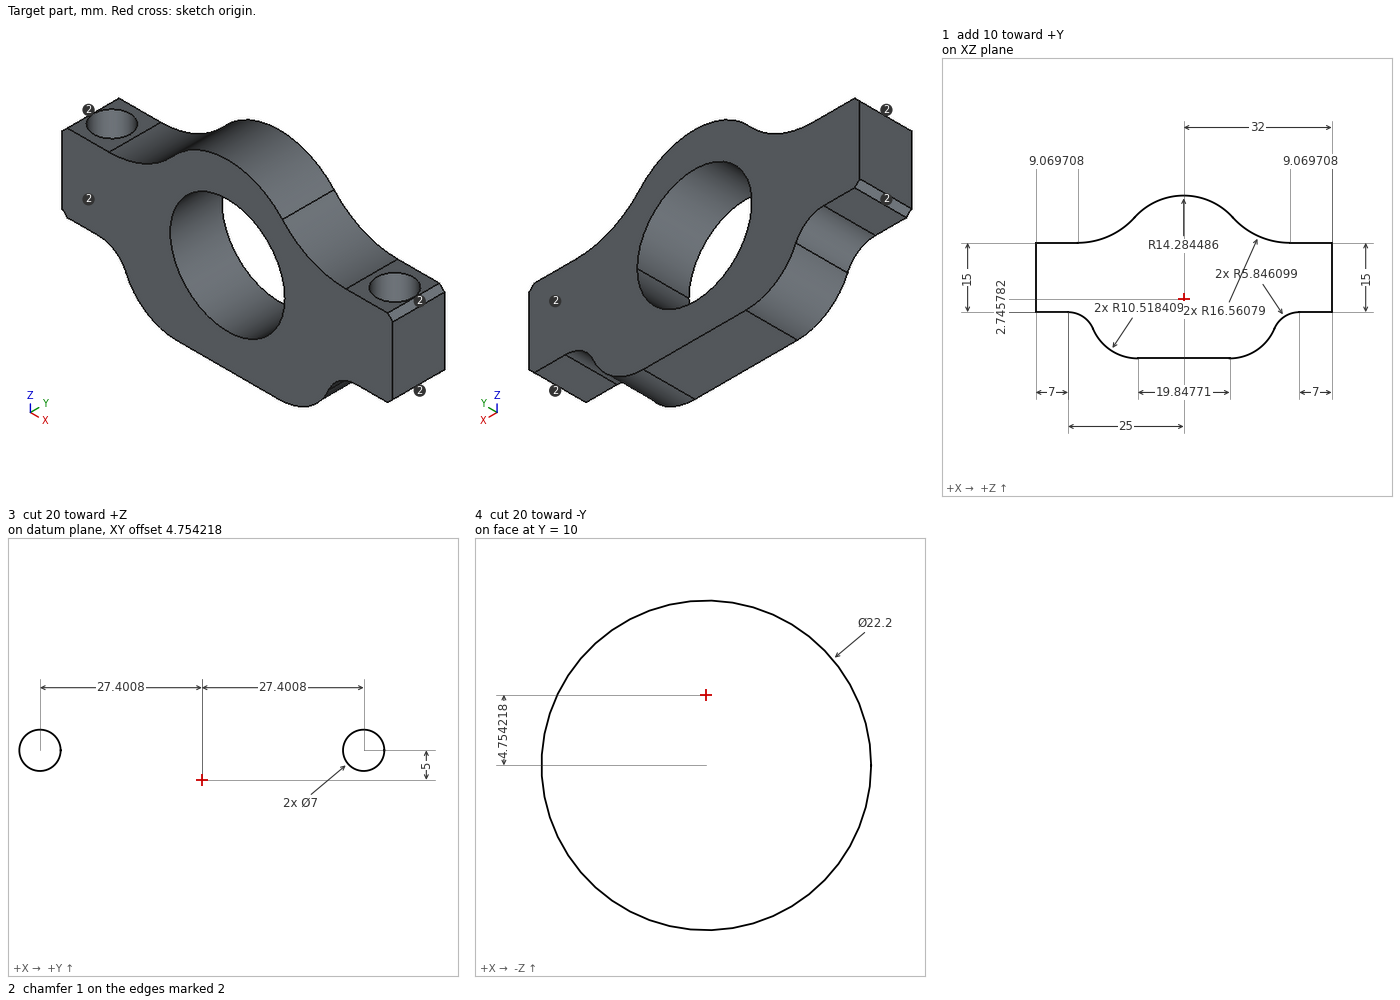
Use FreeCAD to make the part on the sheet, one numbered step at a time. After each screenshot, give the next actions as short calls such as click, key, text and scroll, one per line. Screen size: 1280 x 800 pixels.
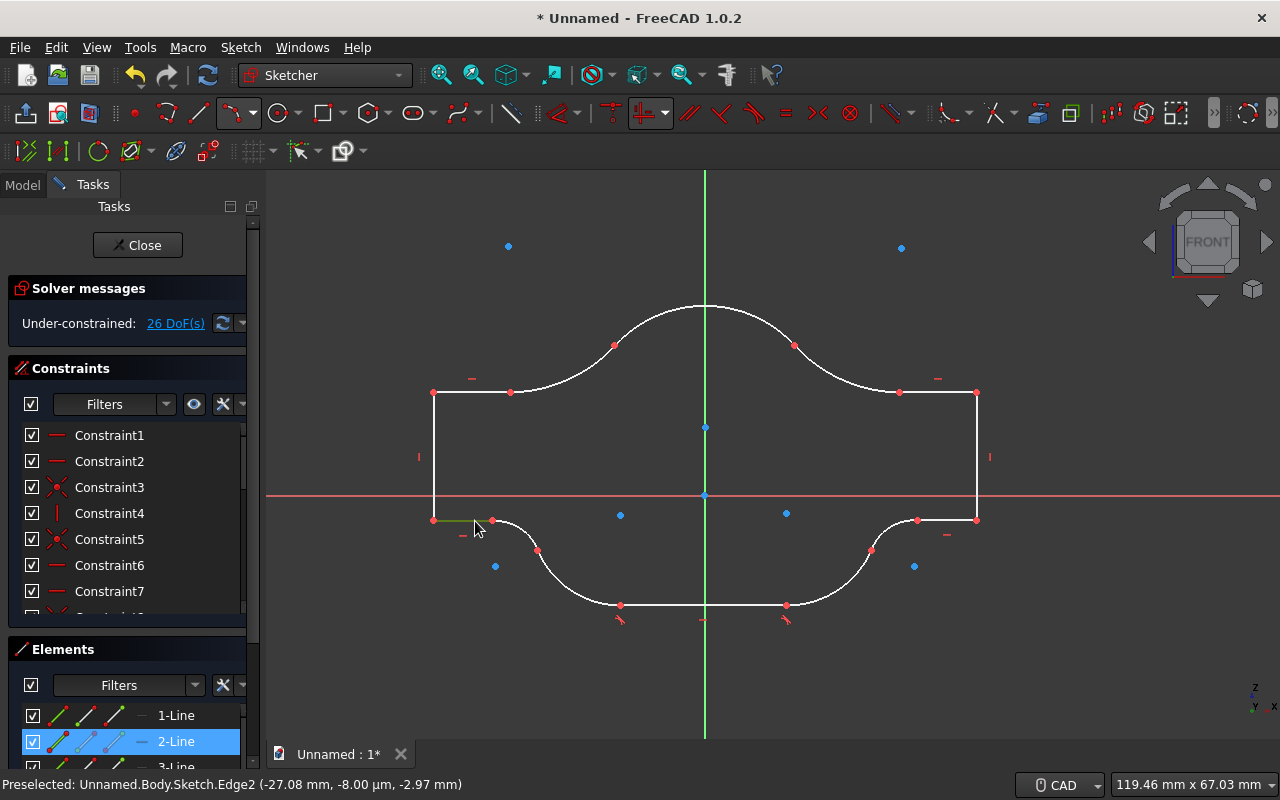
click(529, 536)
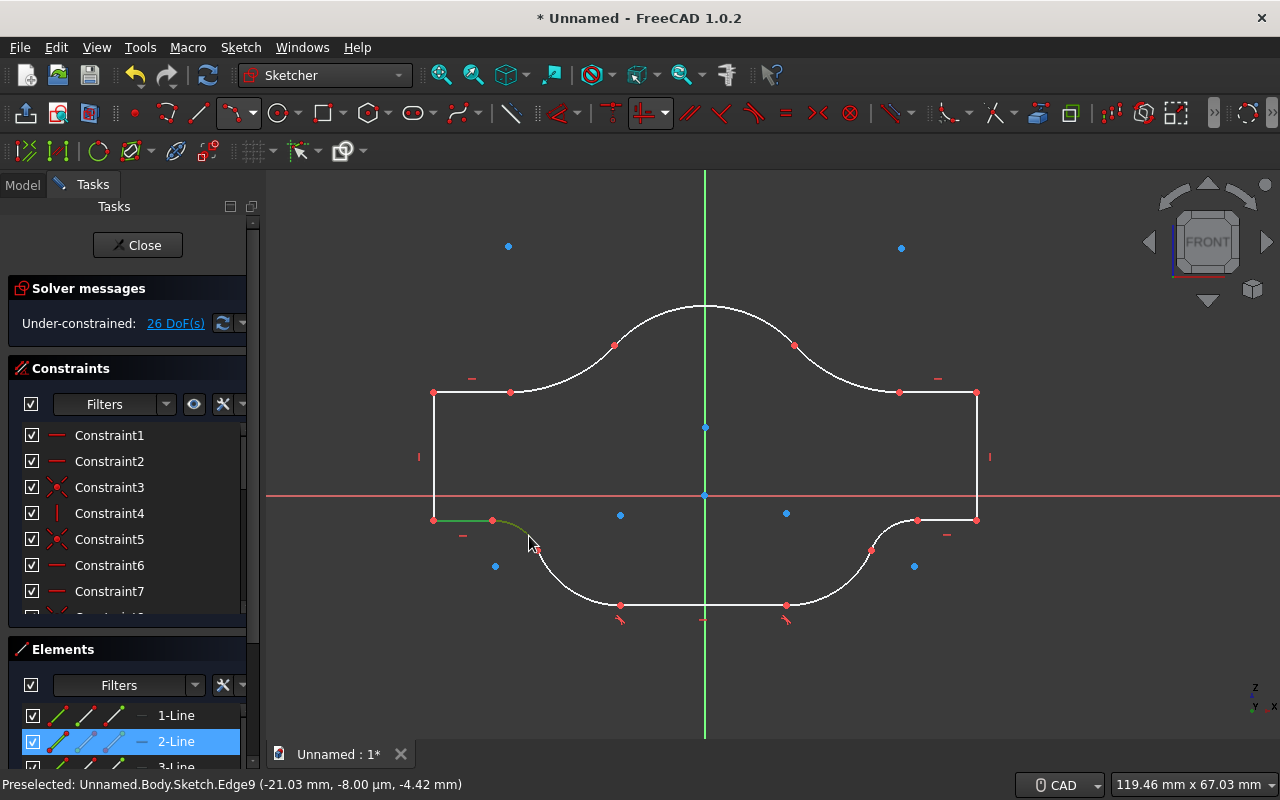
click(754, 114)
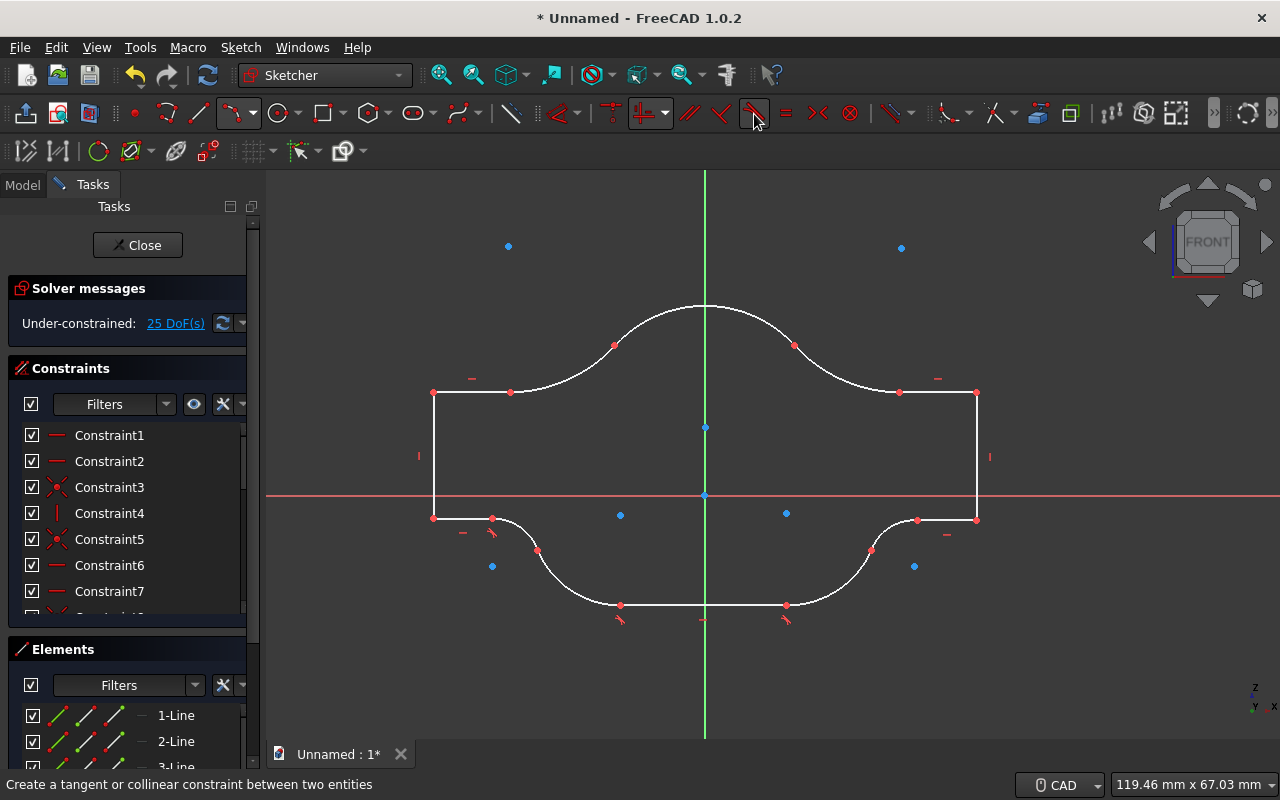
click(457, 392)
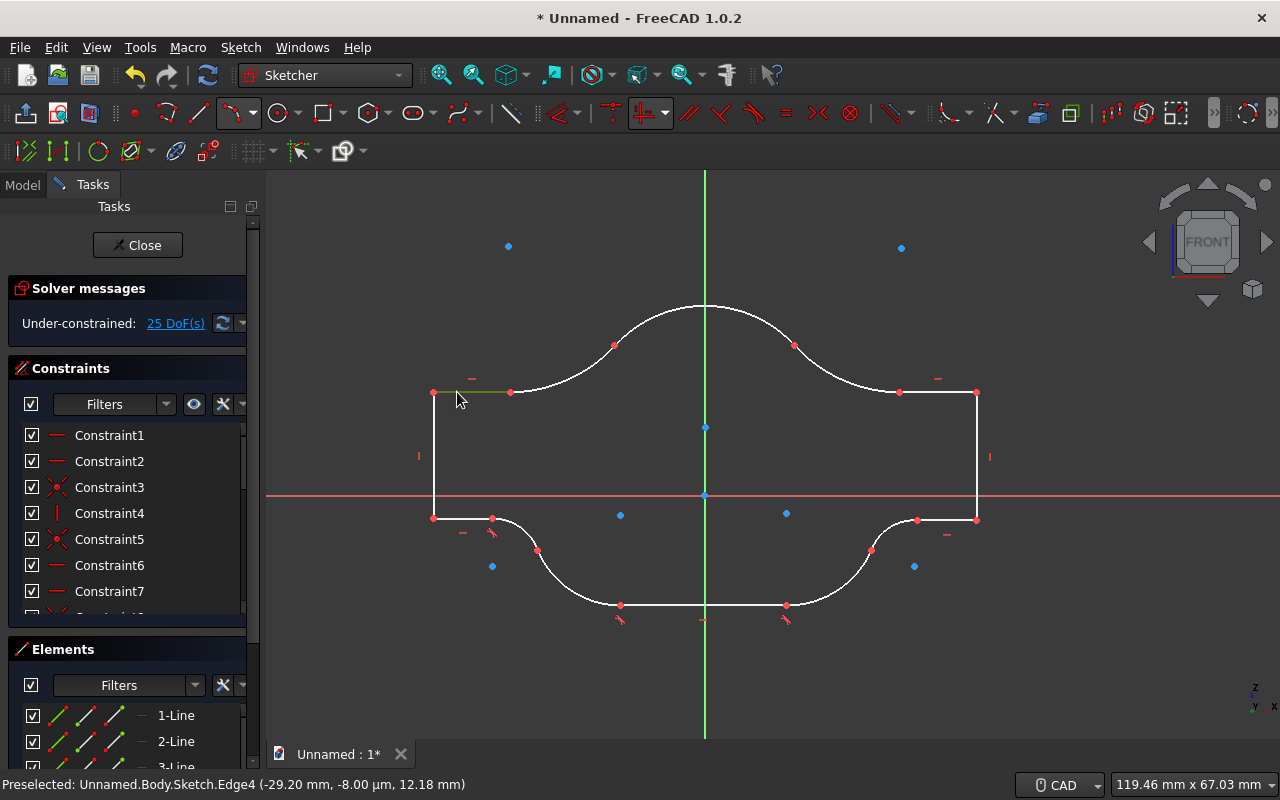
click(545, 388)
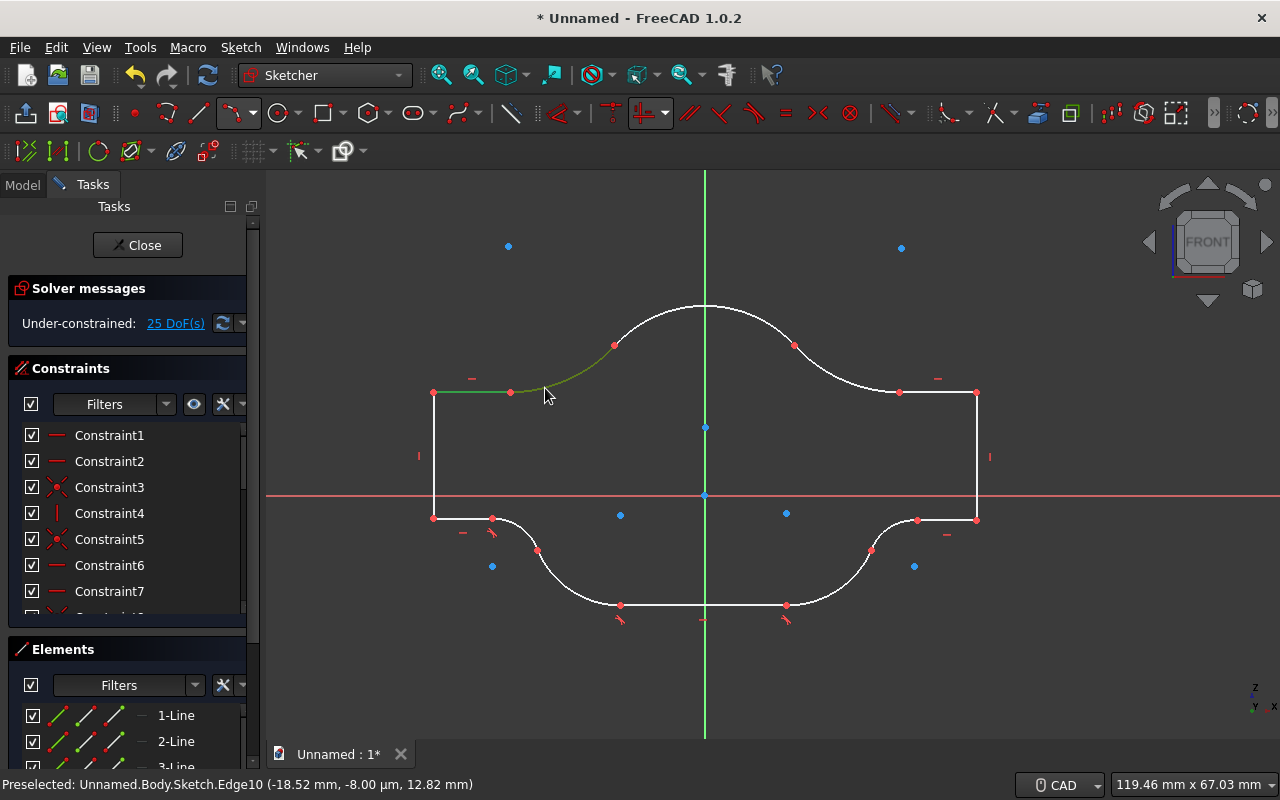
click(754, 114)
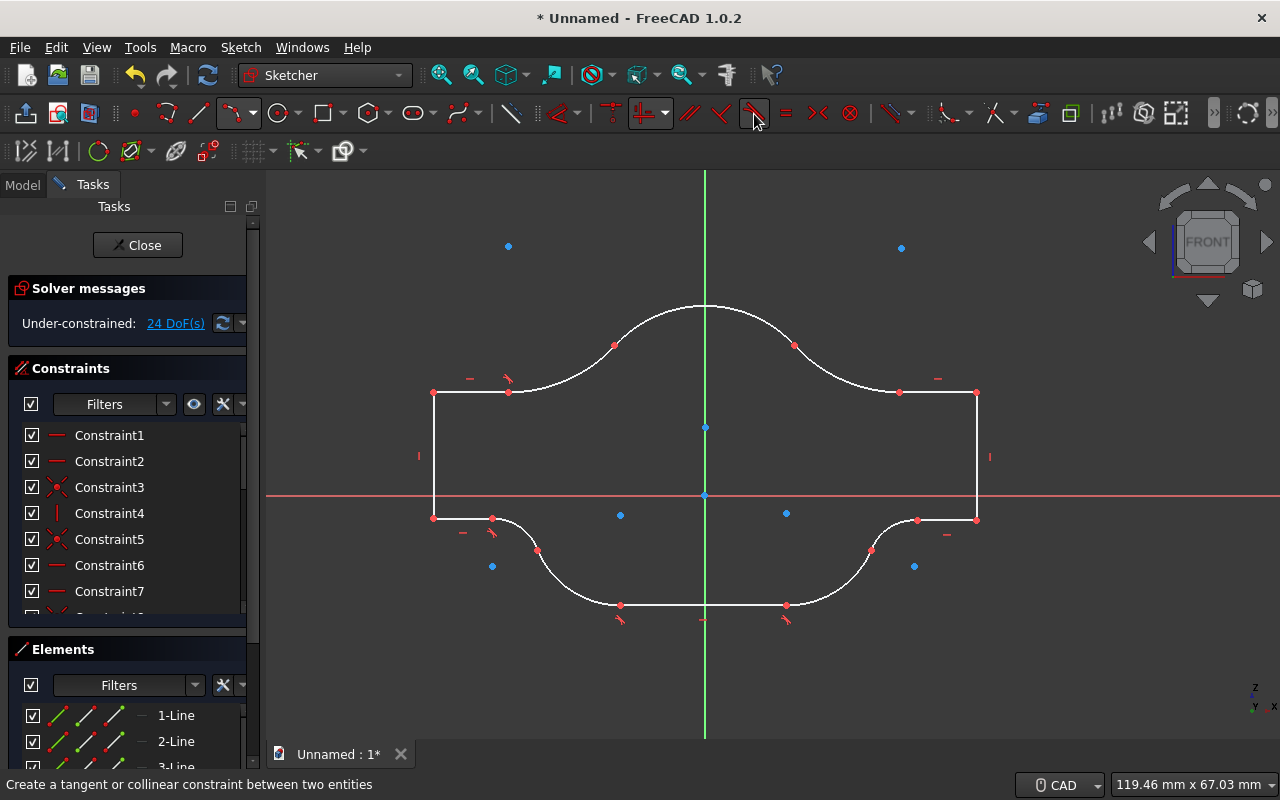
click(923, 392)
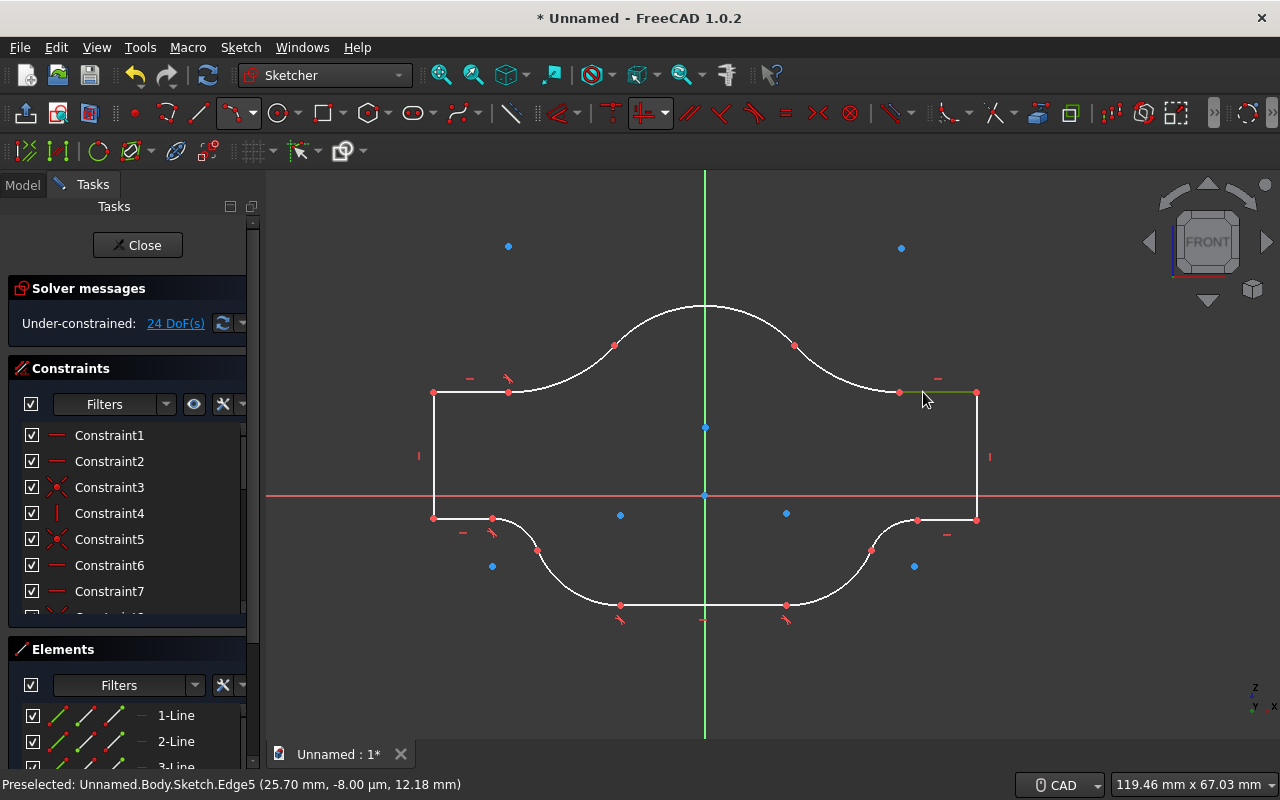
click(822, 369)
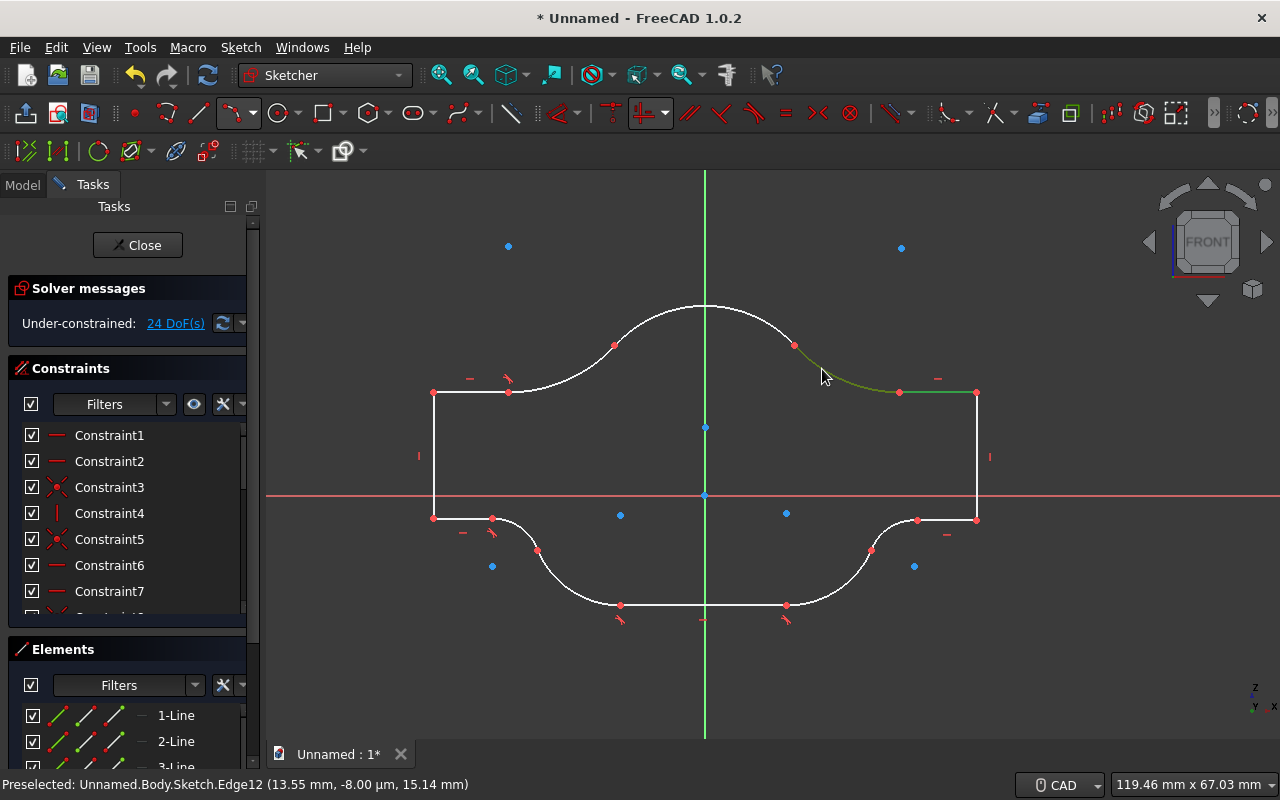
click(754, 114)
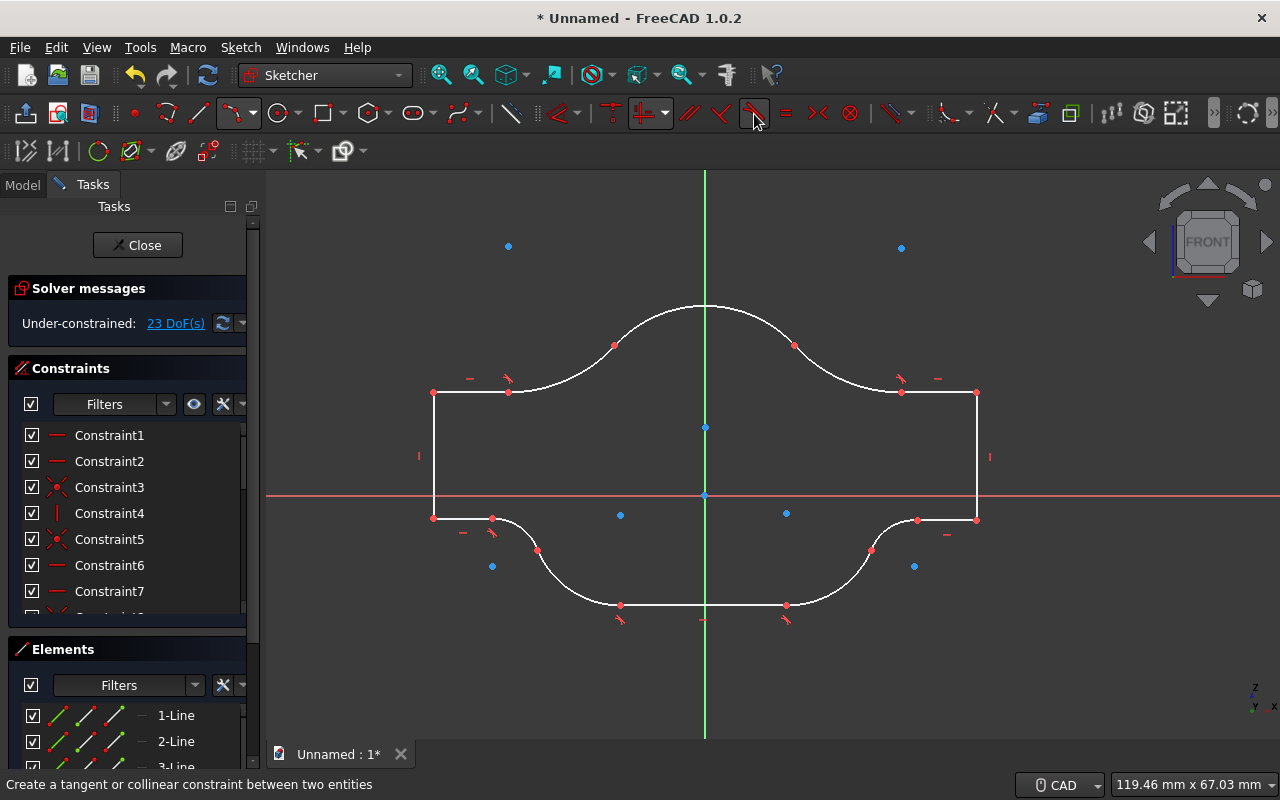
click(959, 520)